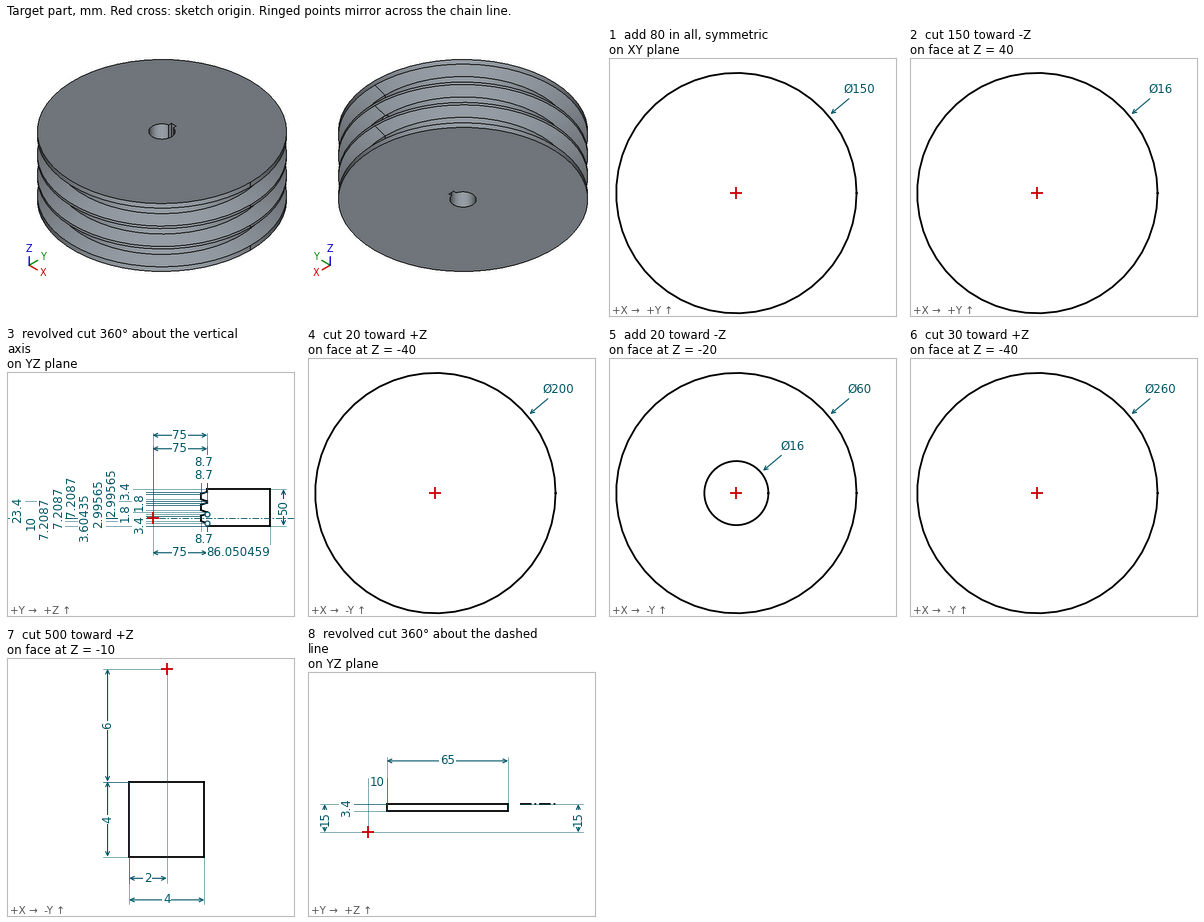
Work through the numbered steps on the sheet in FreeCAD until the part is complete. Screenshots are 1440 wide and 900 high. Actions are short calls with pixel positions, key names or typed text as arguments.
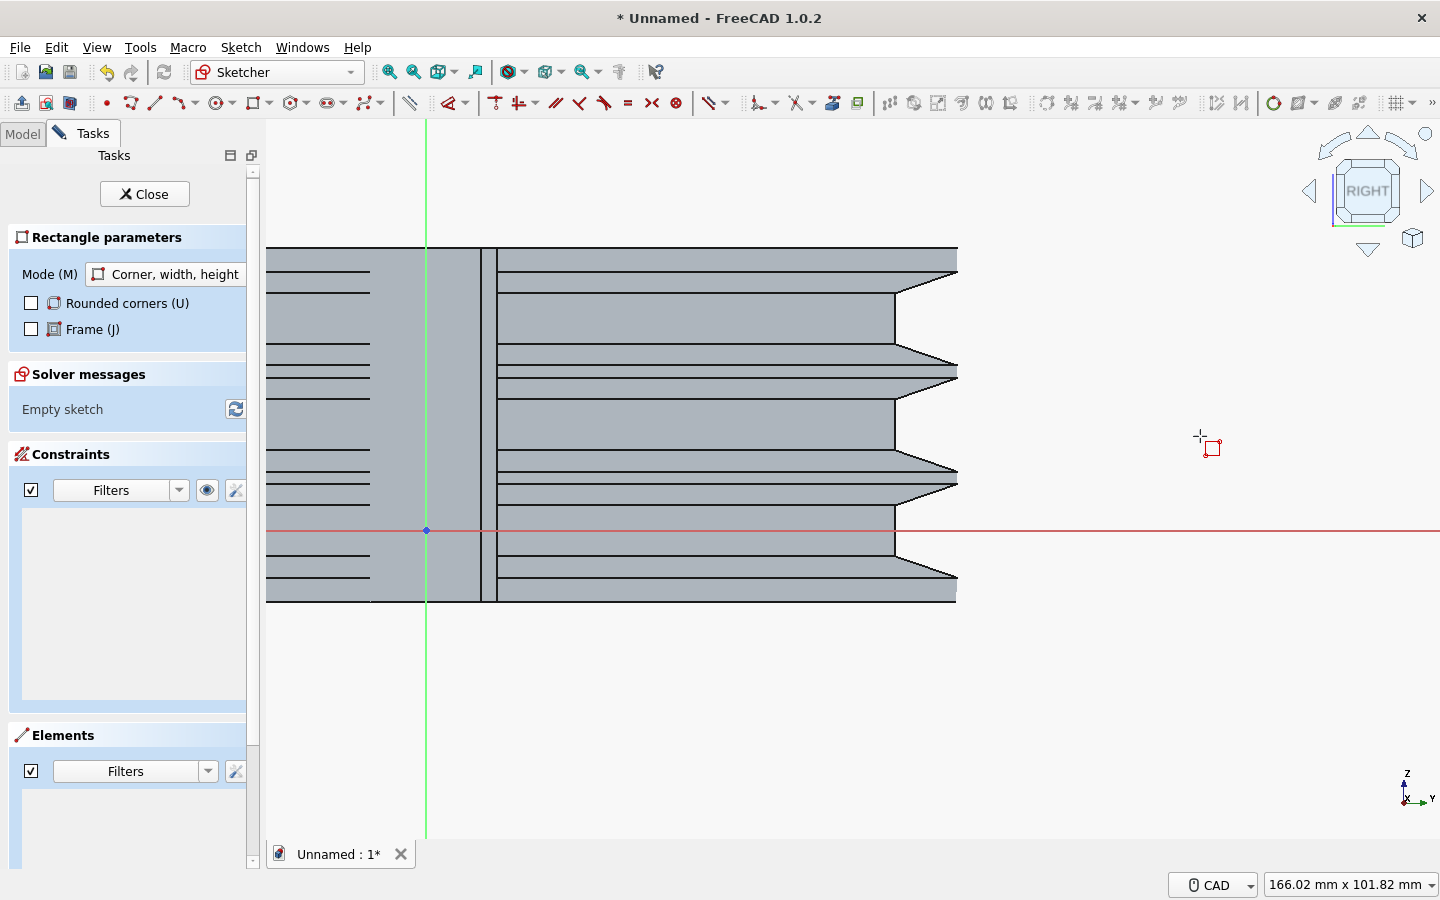
click(497, 425)
click(957, 449)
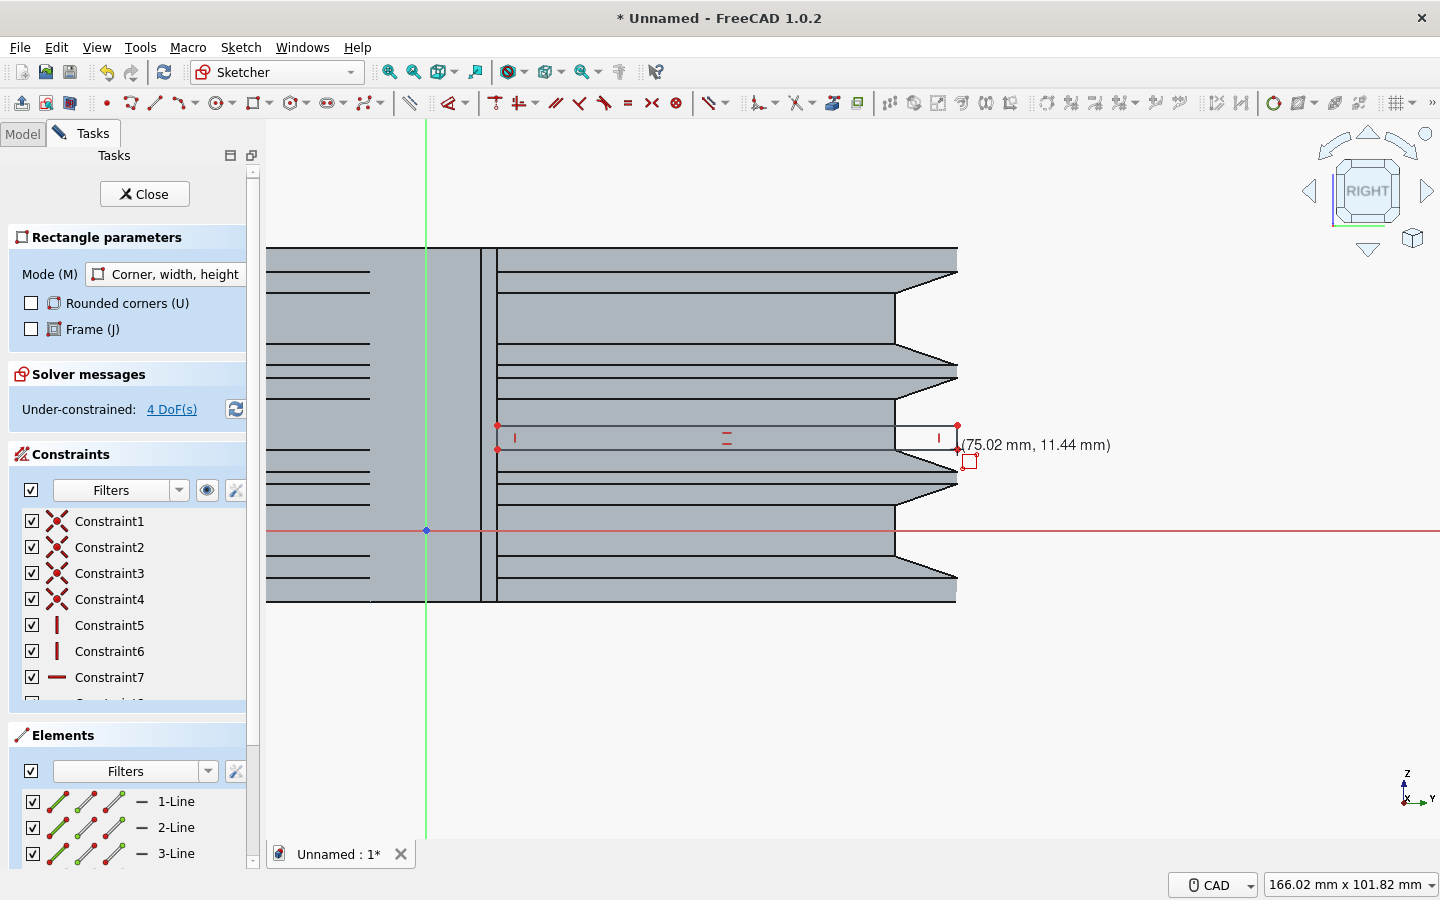
key(g)
key(l)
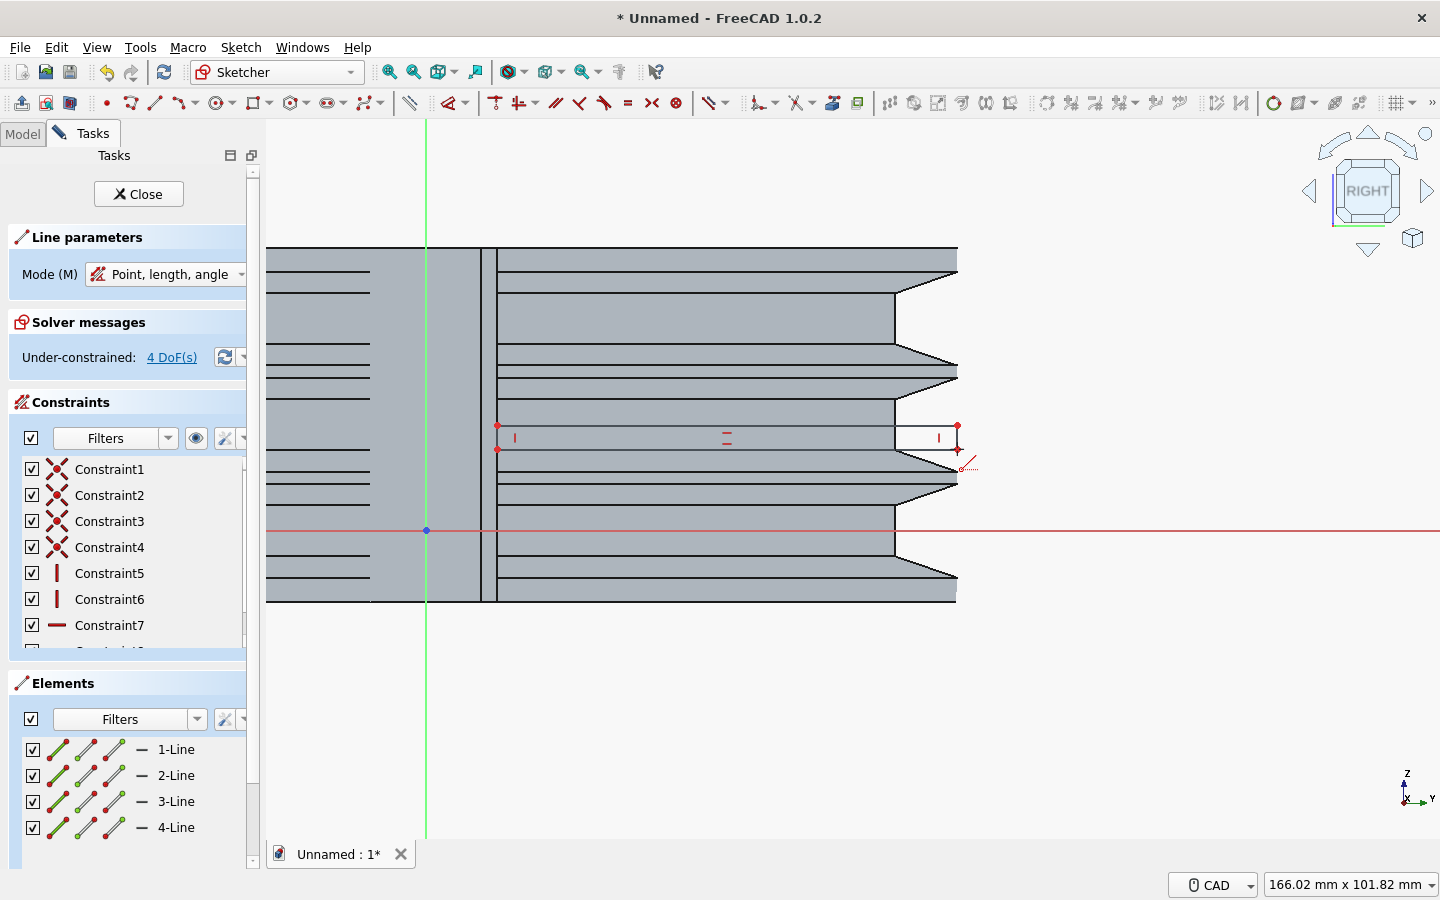
click(1003, 425)
click(1141, 425)
key(Escape)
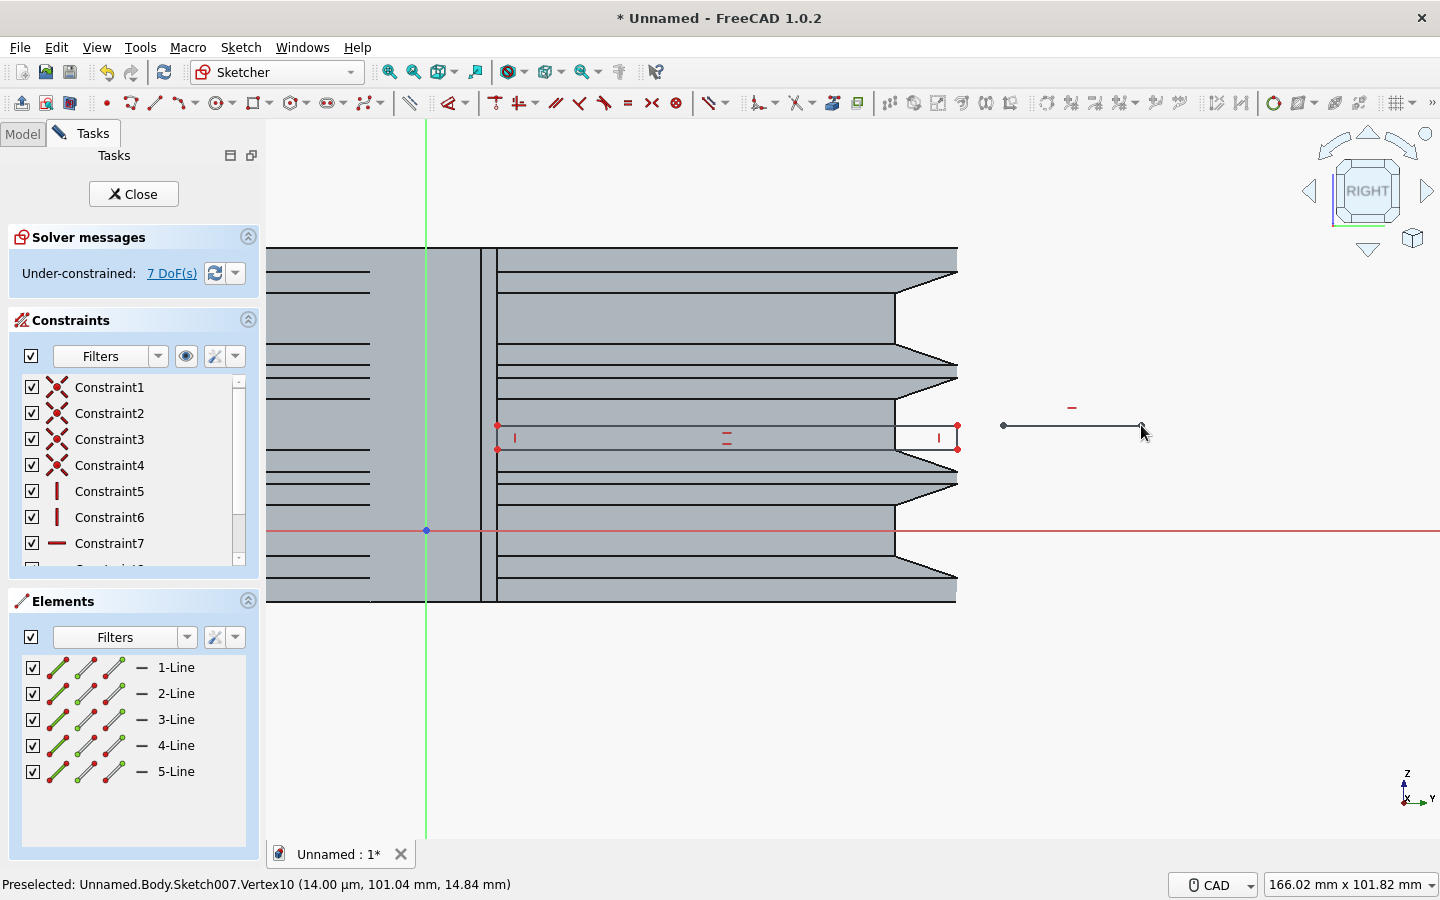
click(1044, 426)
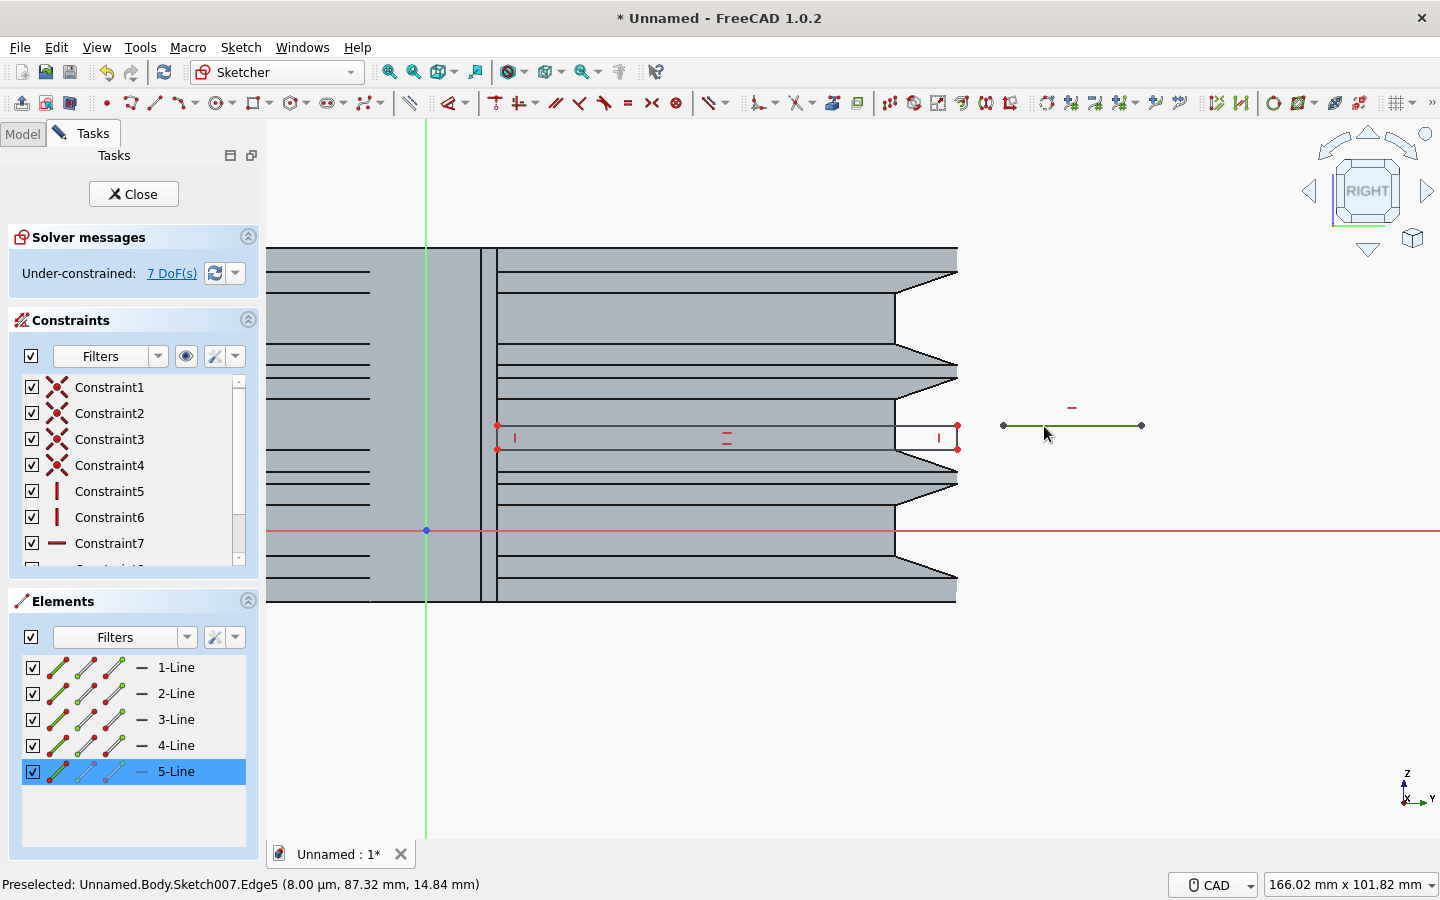
key(g)
key(n)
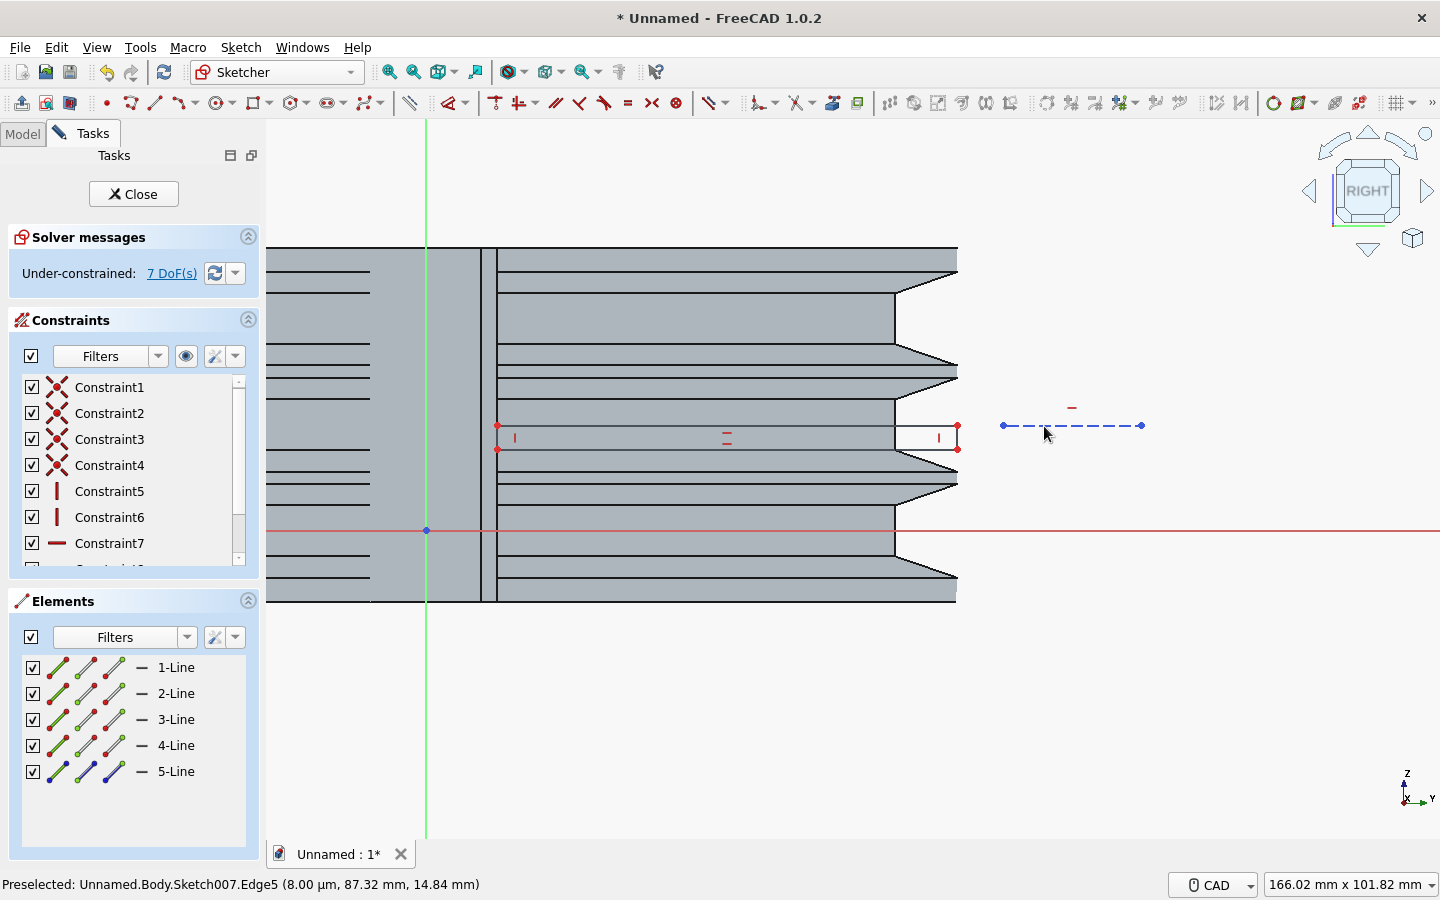
key(d)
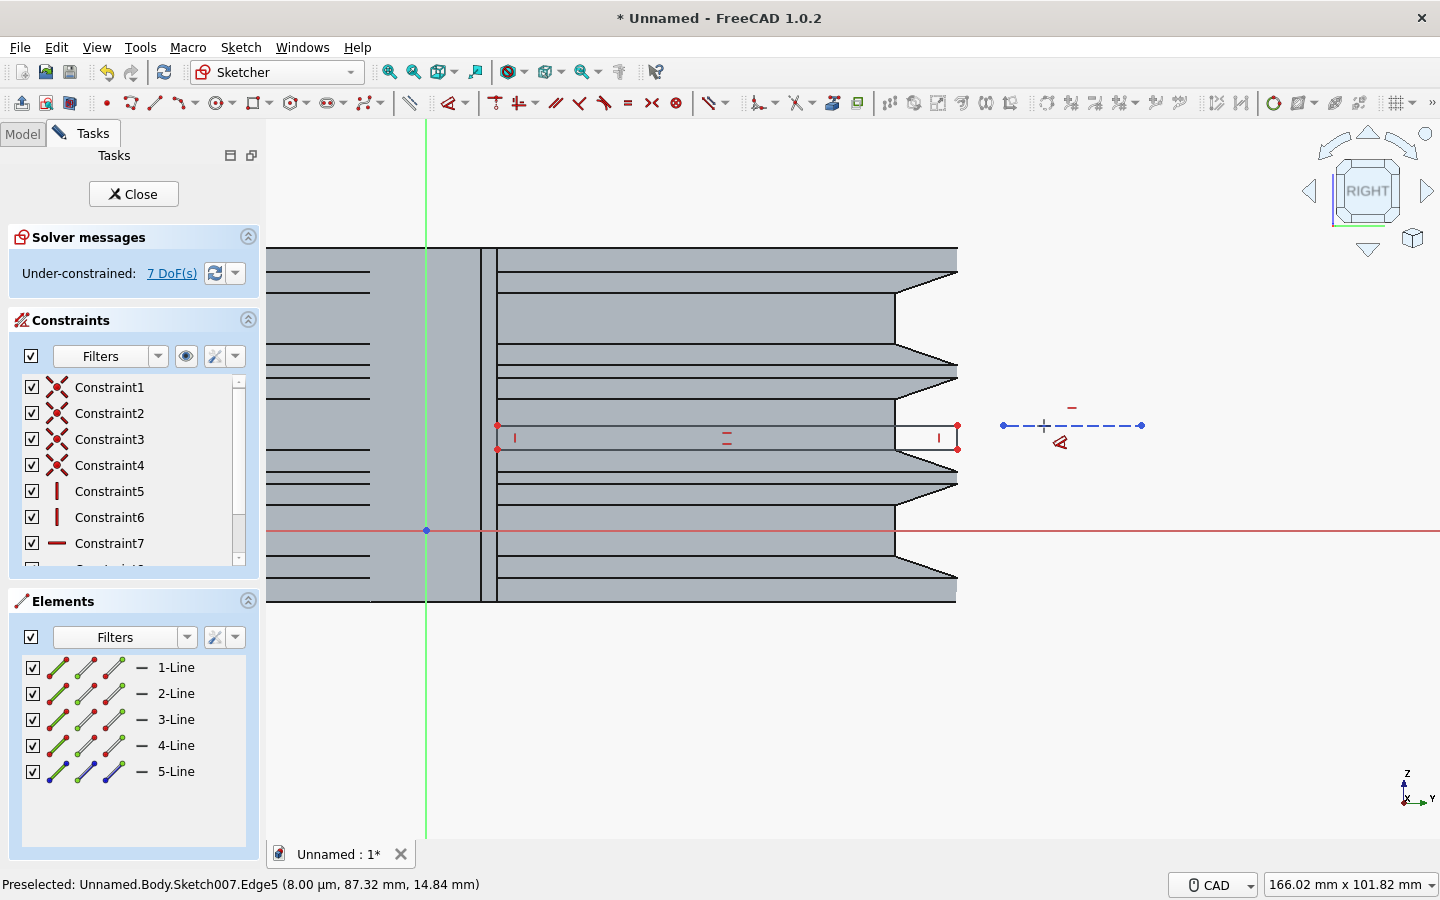
click(635, 450)
click(727, 484)